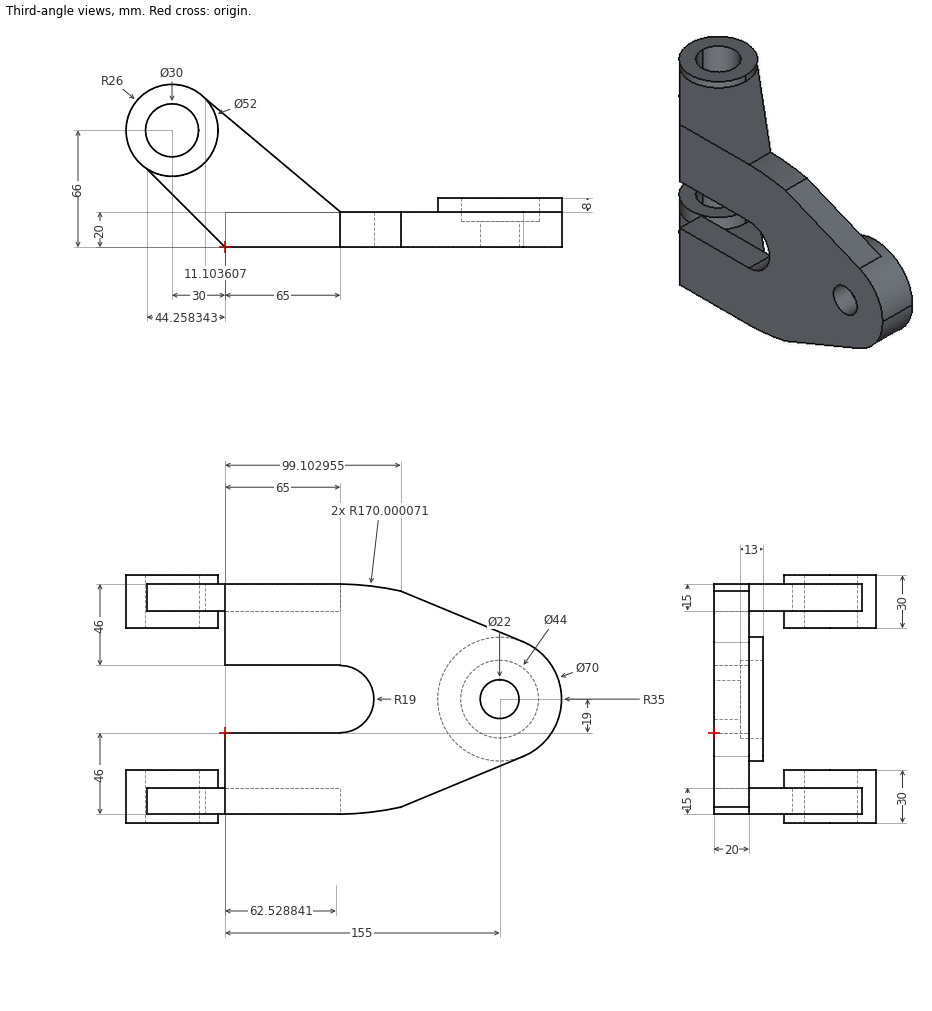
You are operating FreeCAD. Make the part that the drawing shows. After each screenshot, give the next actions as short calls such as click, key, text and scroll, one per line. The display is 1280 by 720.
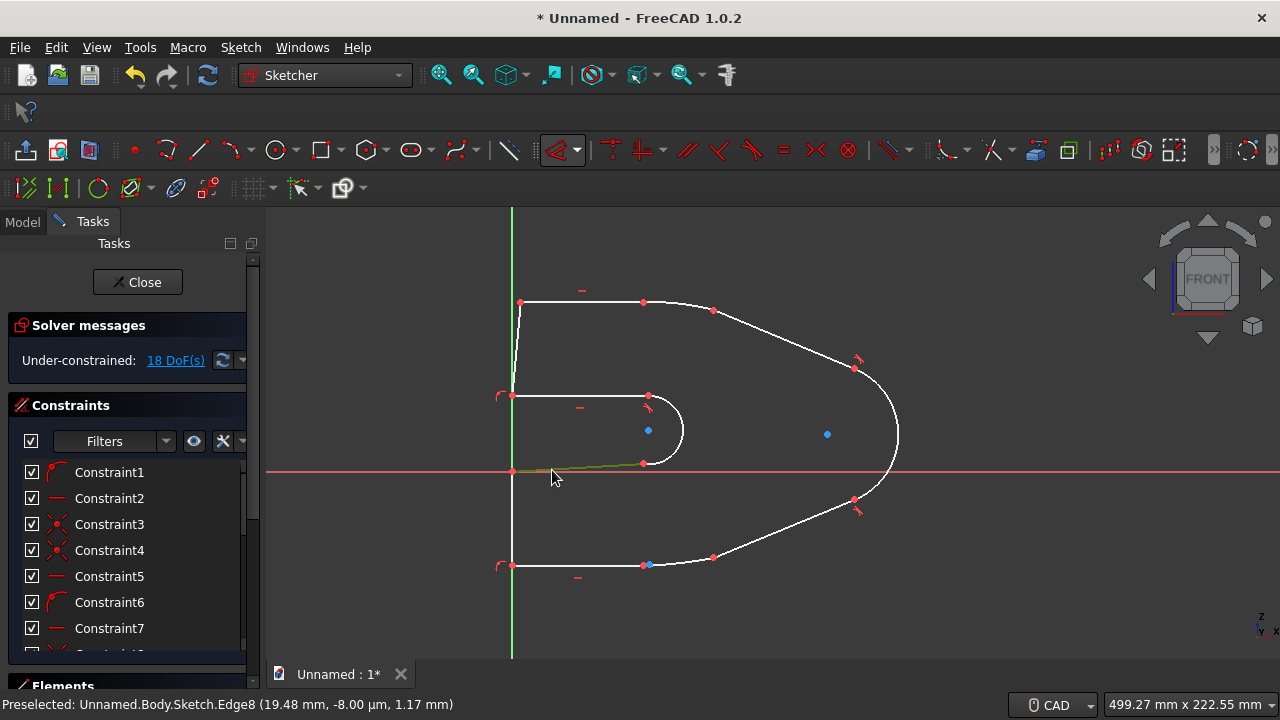
click(674, 453)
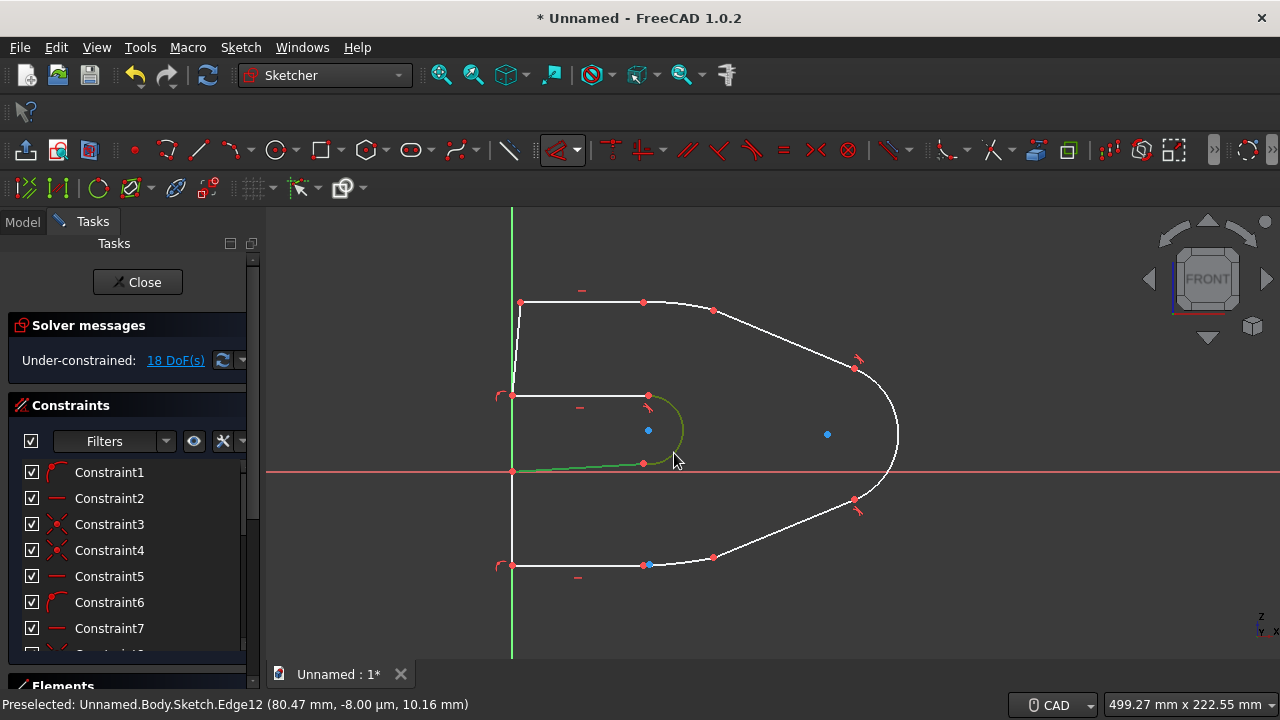
key(t)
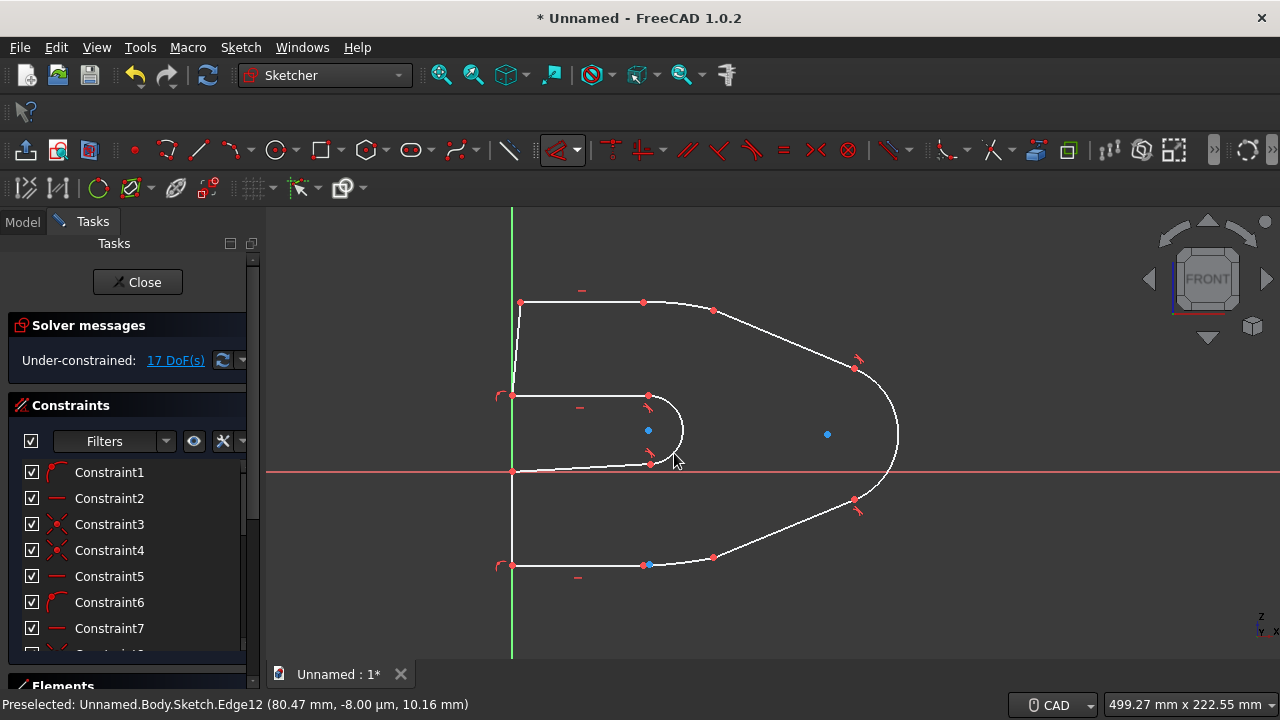
click(515, 368)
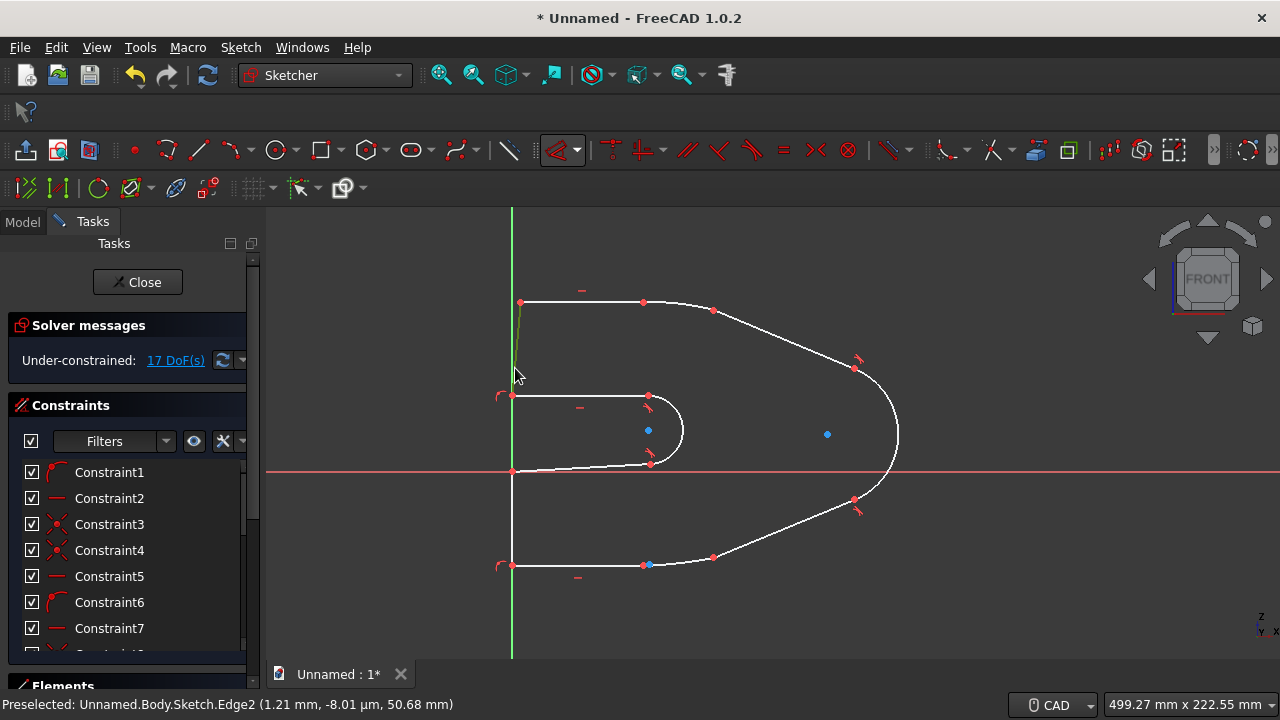
key(v)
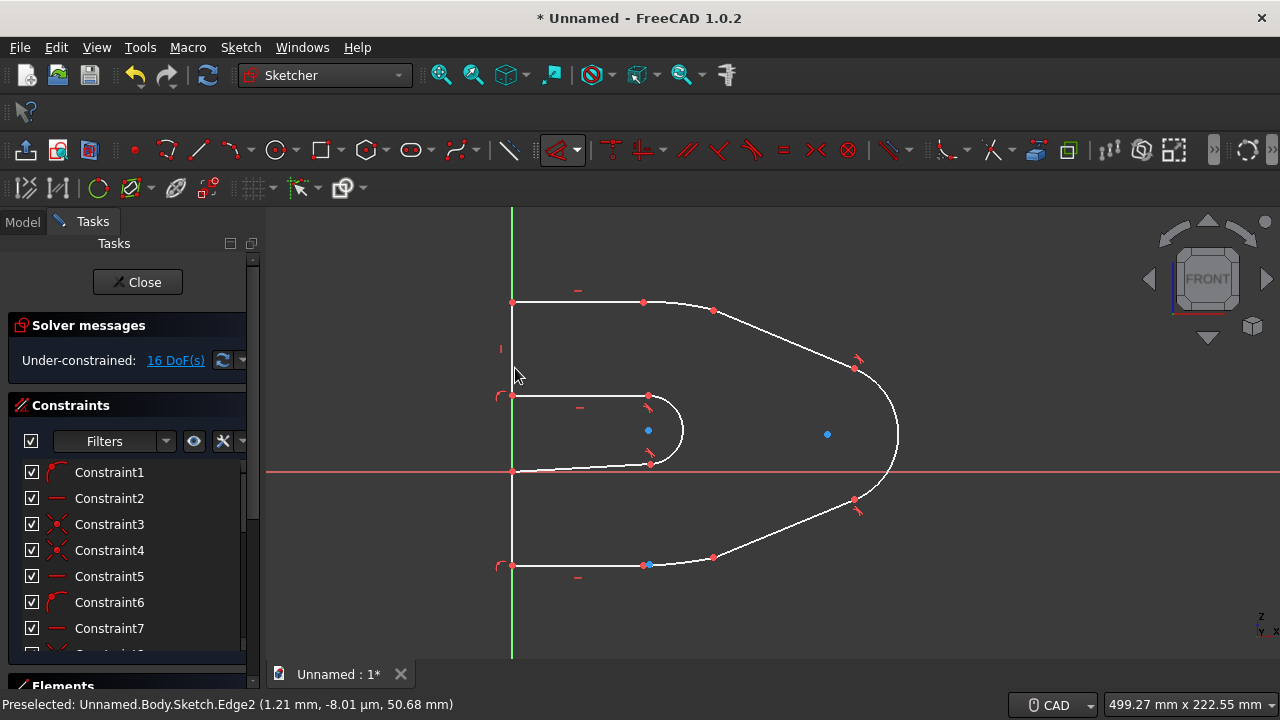
click(554, 470)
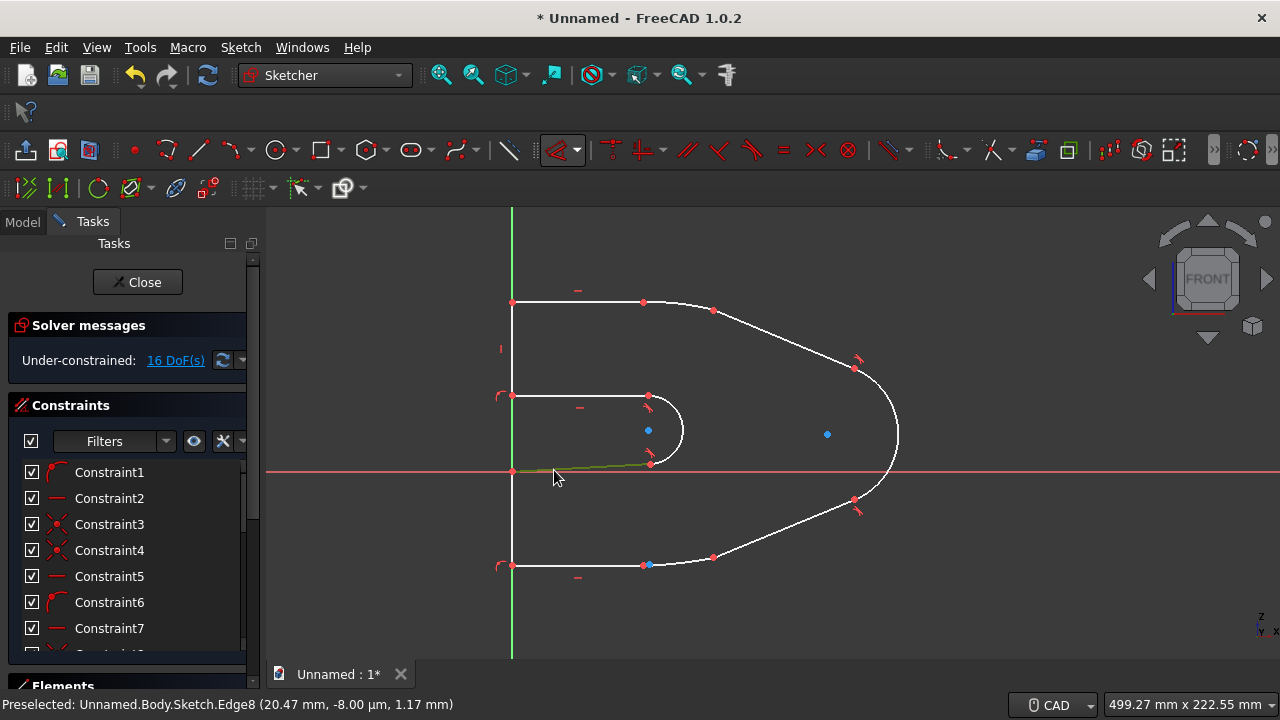
key(h)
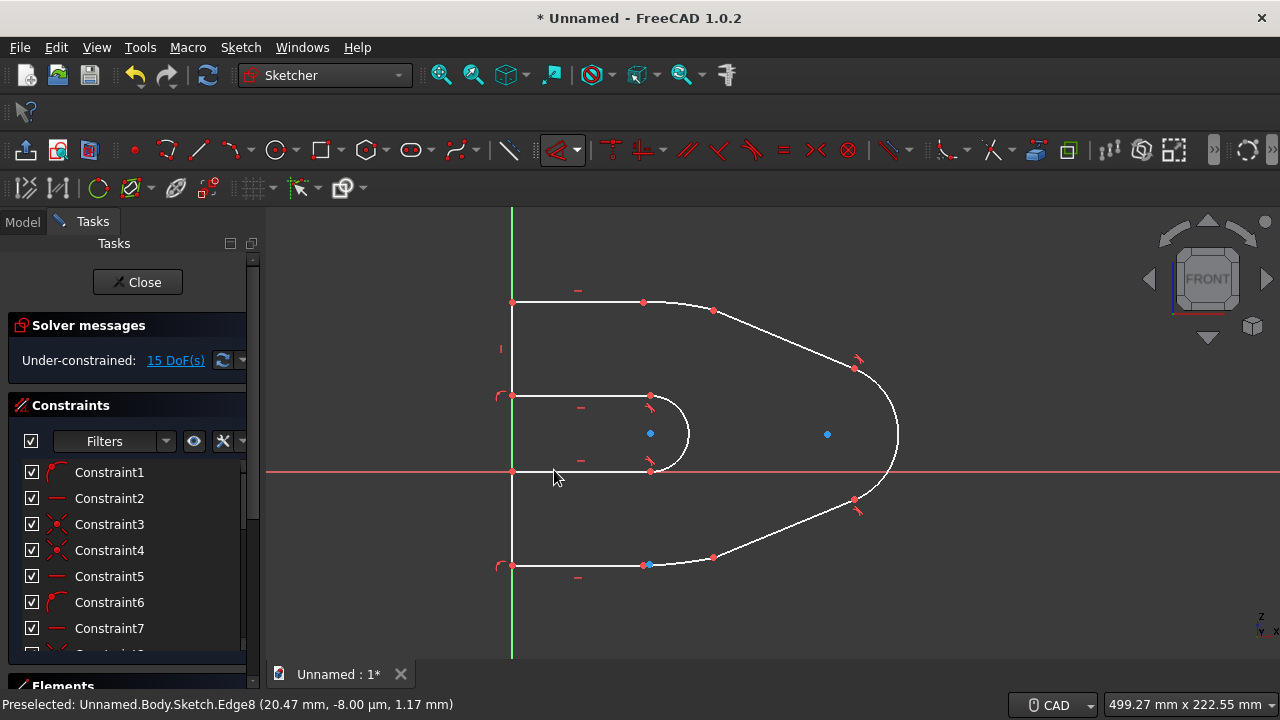
click(693, 306)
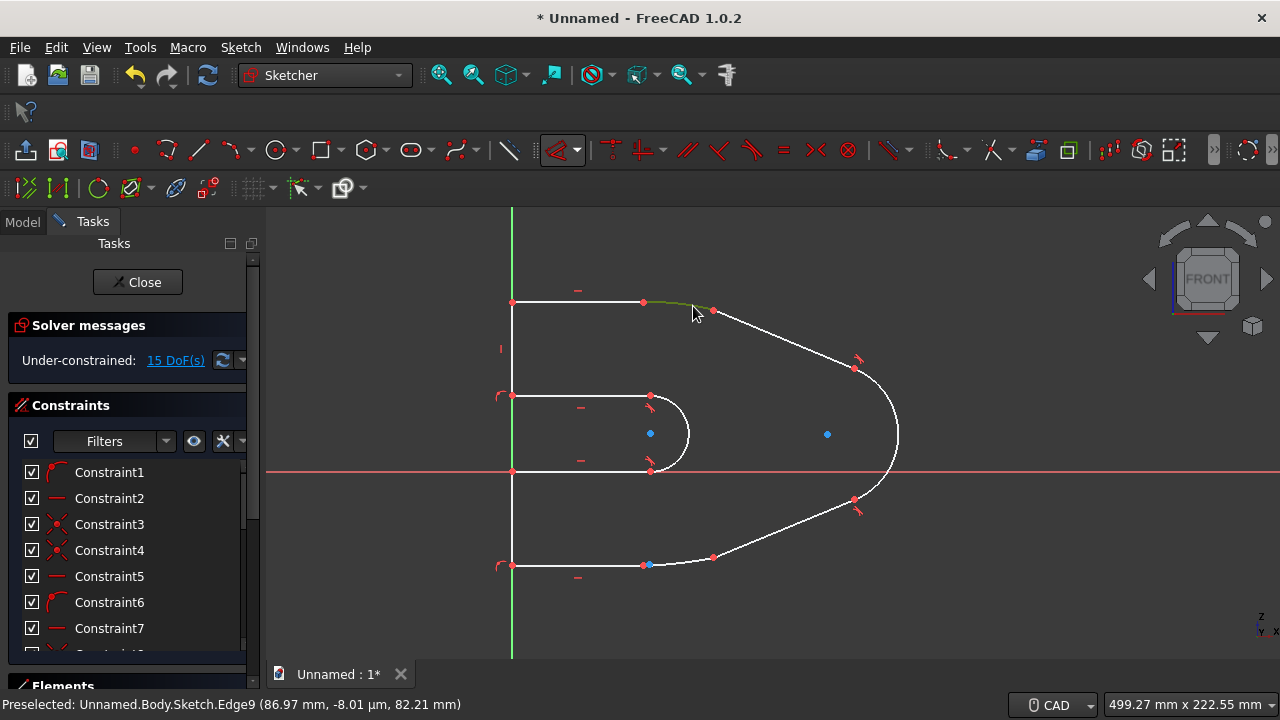
click(665, 565)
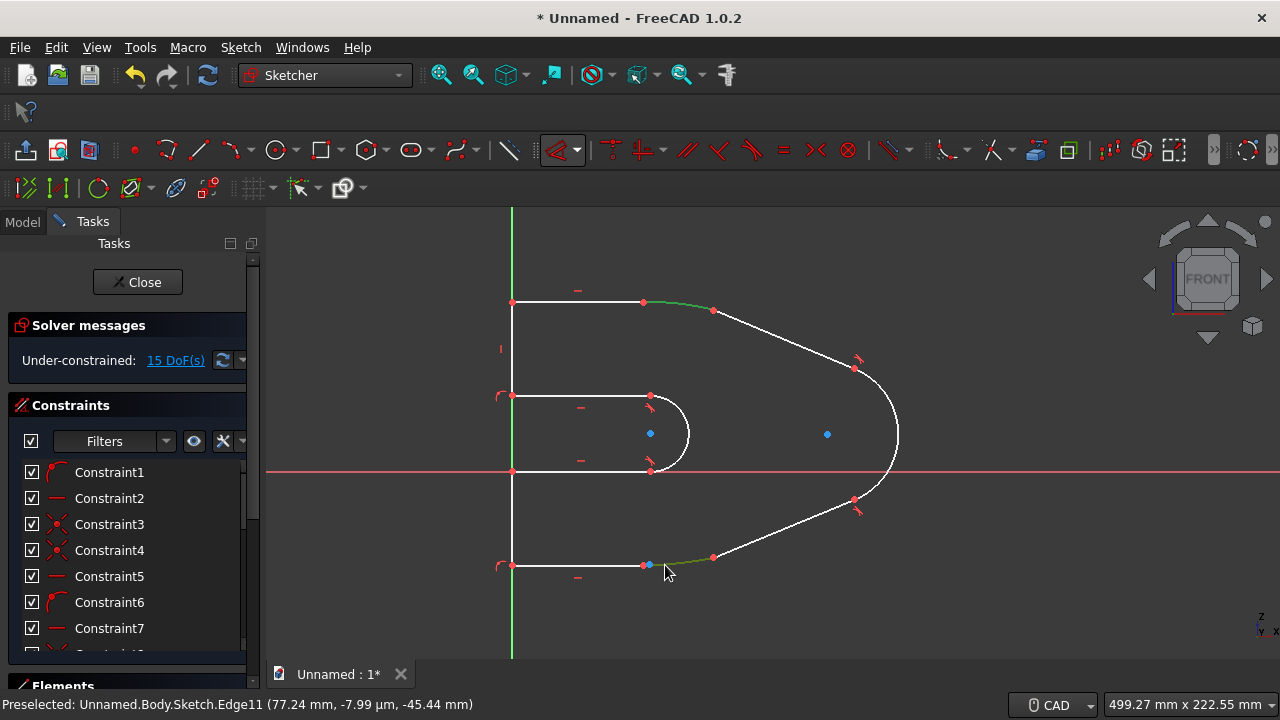
key(e)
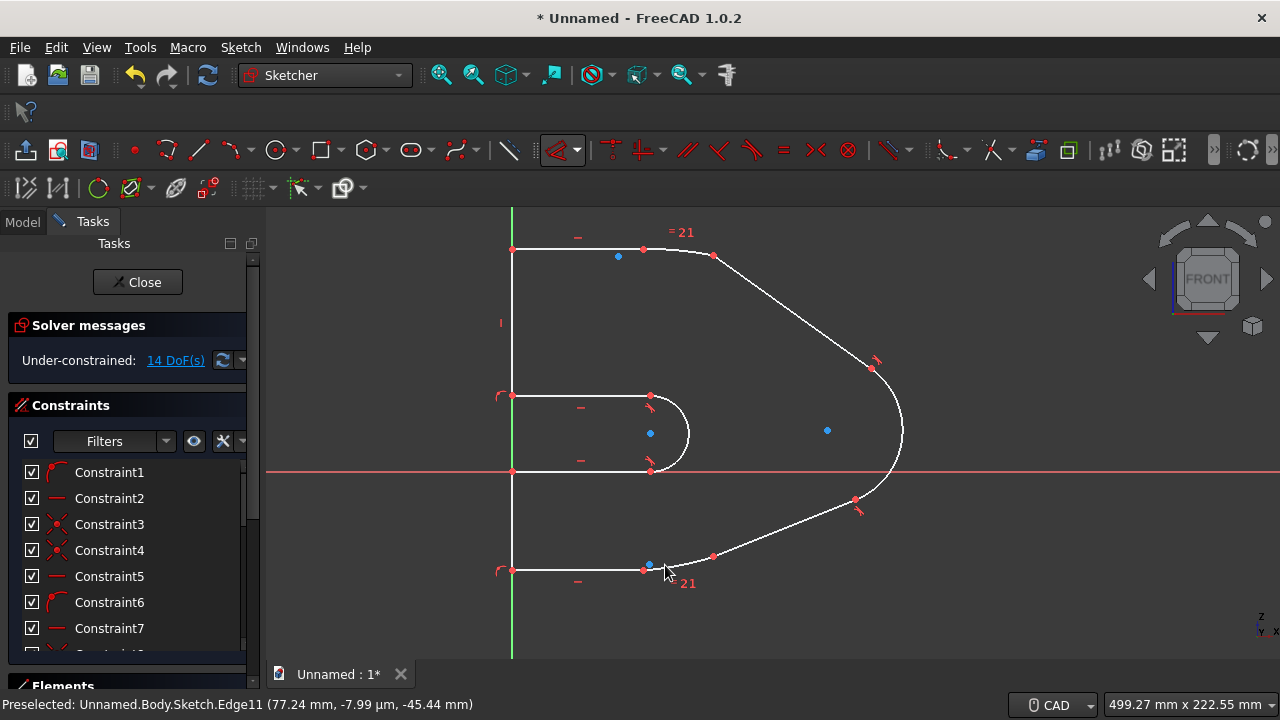
click(556, 150)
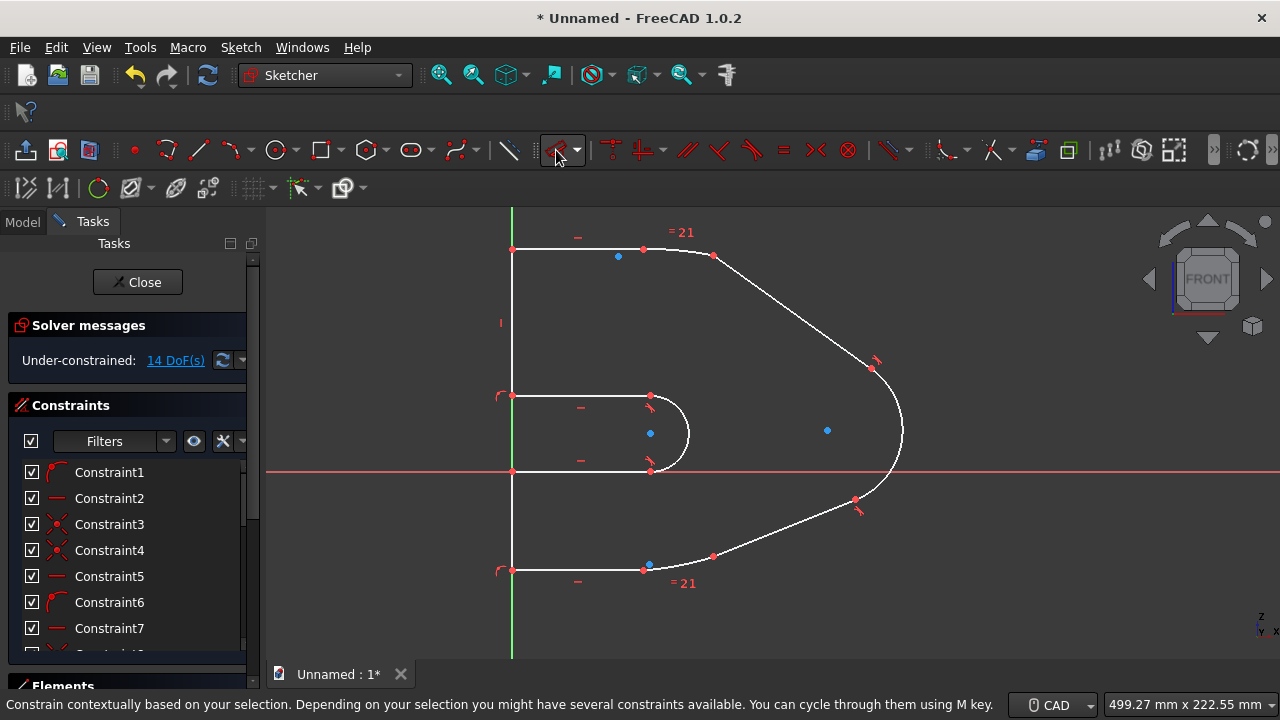
click(693, 252)
click(856, 285)